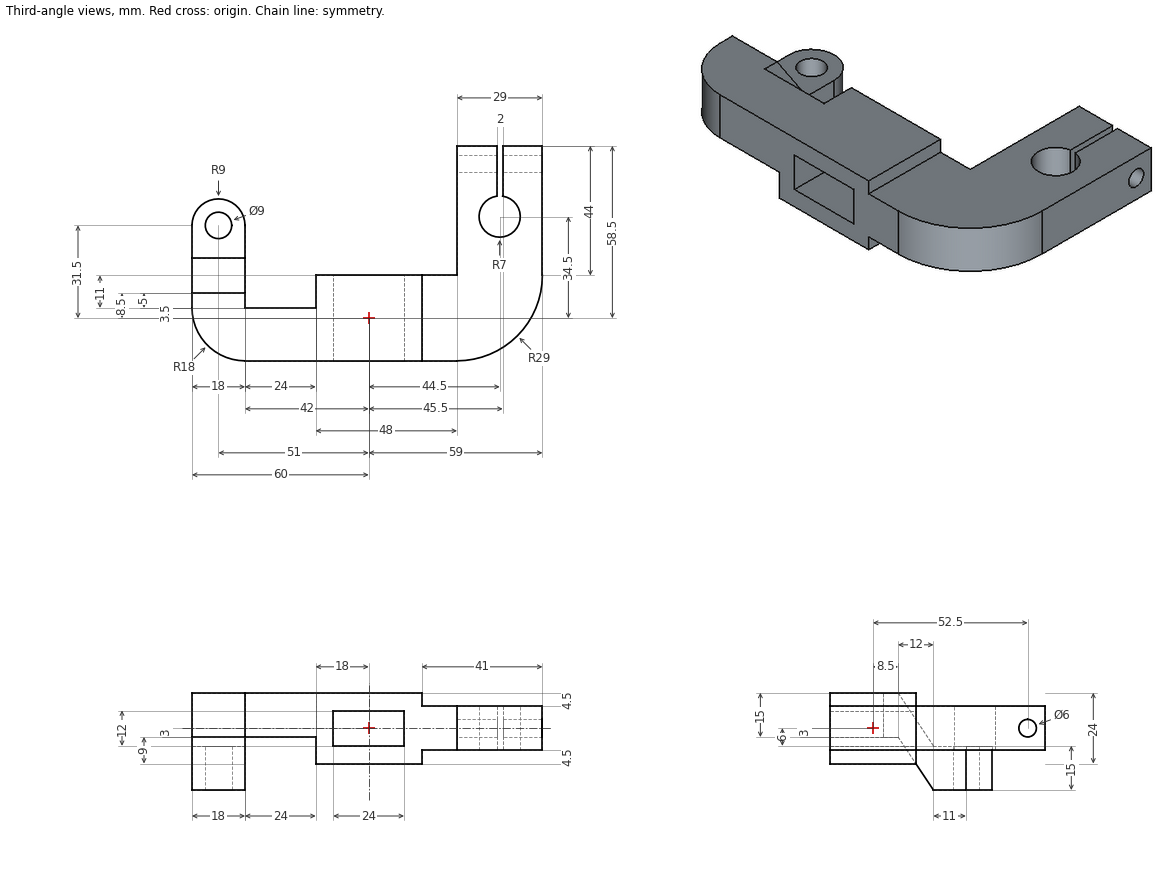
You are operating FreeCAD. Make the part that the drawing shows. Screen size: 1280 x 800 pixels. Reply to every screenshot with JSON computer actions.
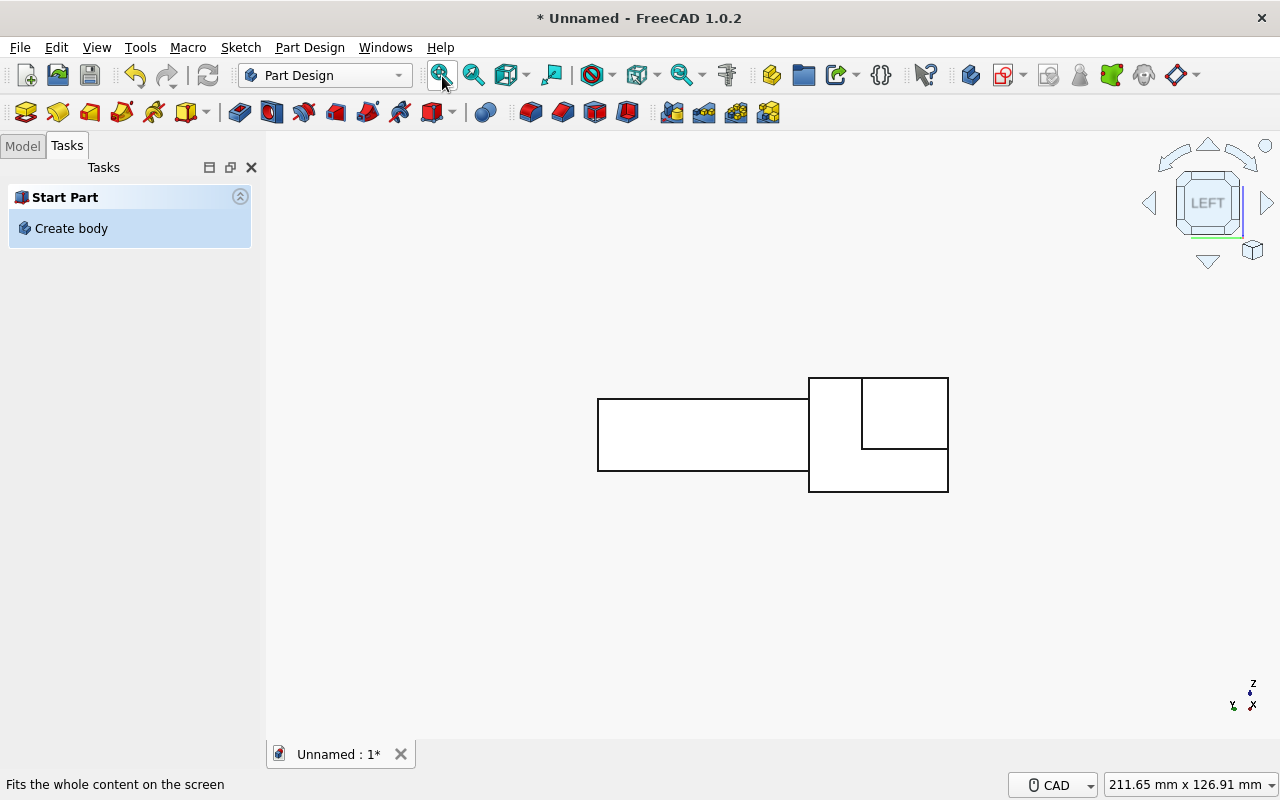
{"action": "left_click", "coordinate": [673, 434]}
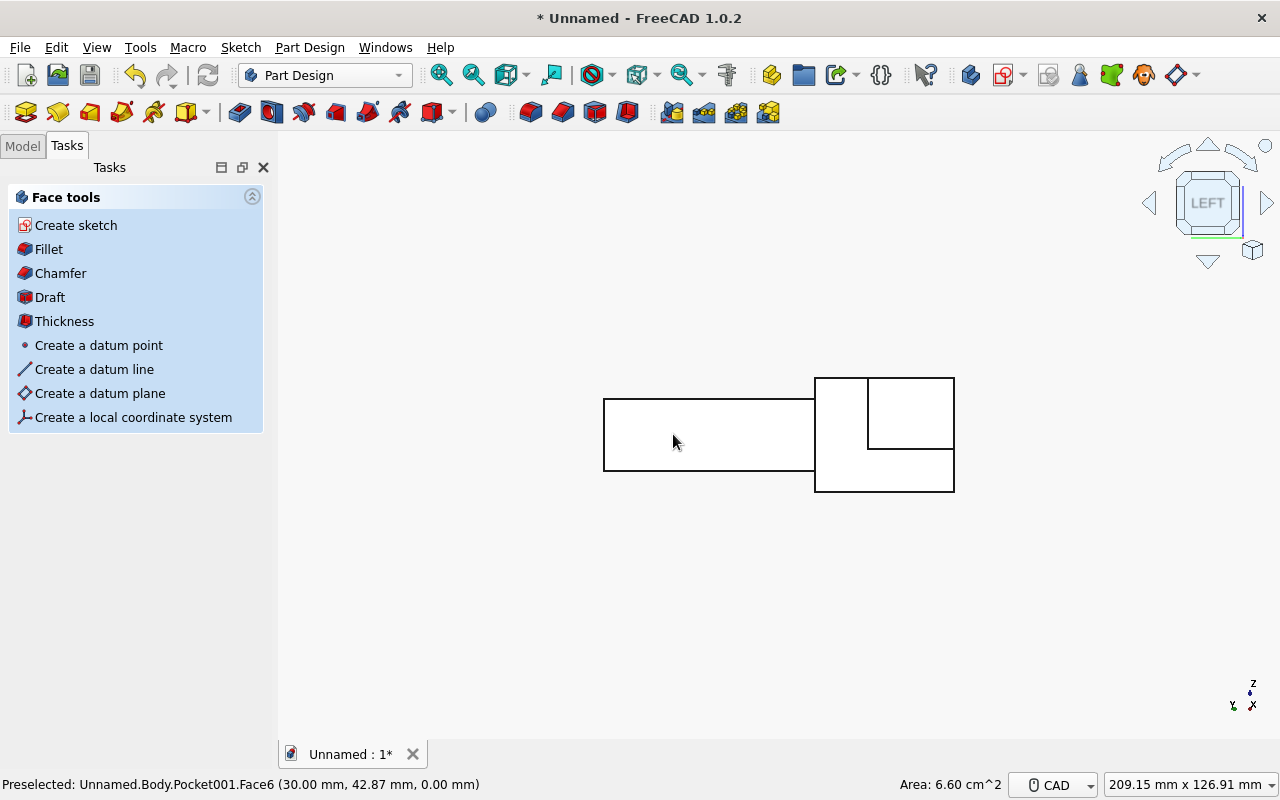
{"action": "left_click", "coordinate": [1004, 76]}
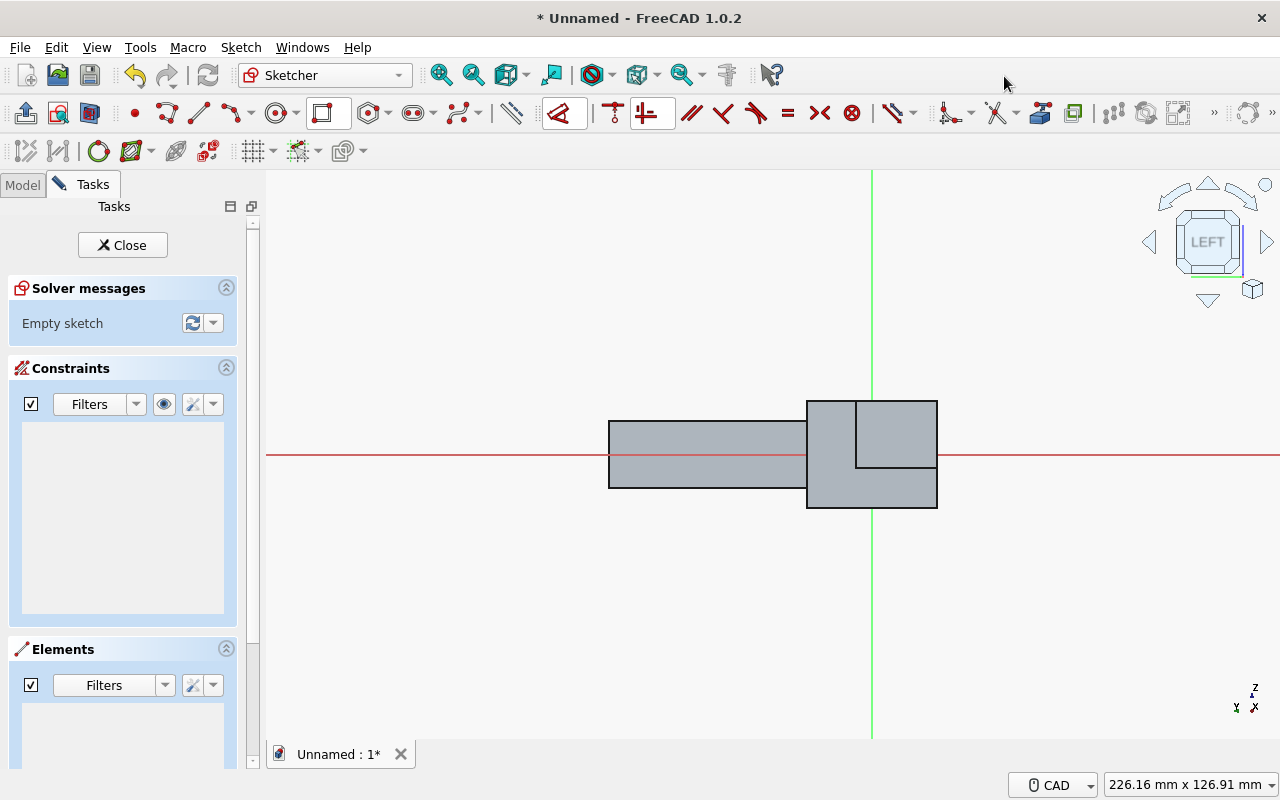
{"action": "scroll", "coordinate": [631, 454], "scroll_direction": "up", "scroll_amount": 13}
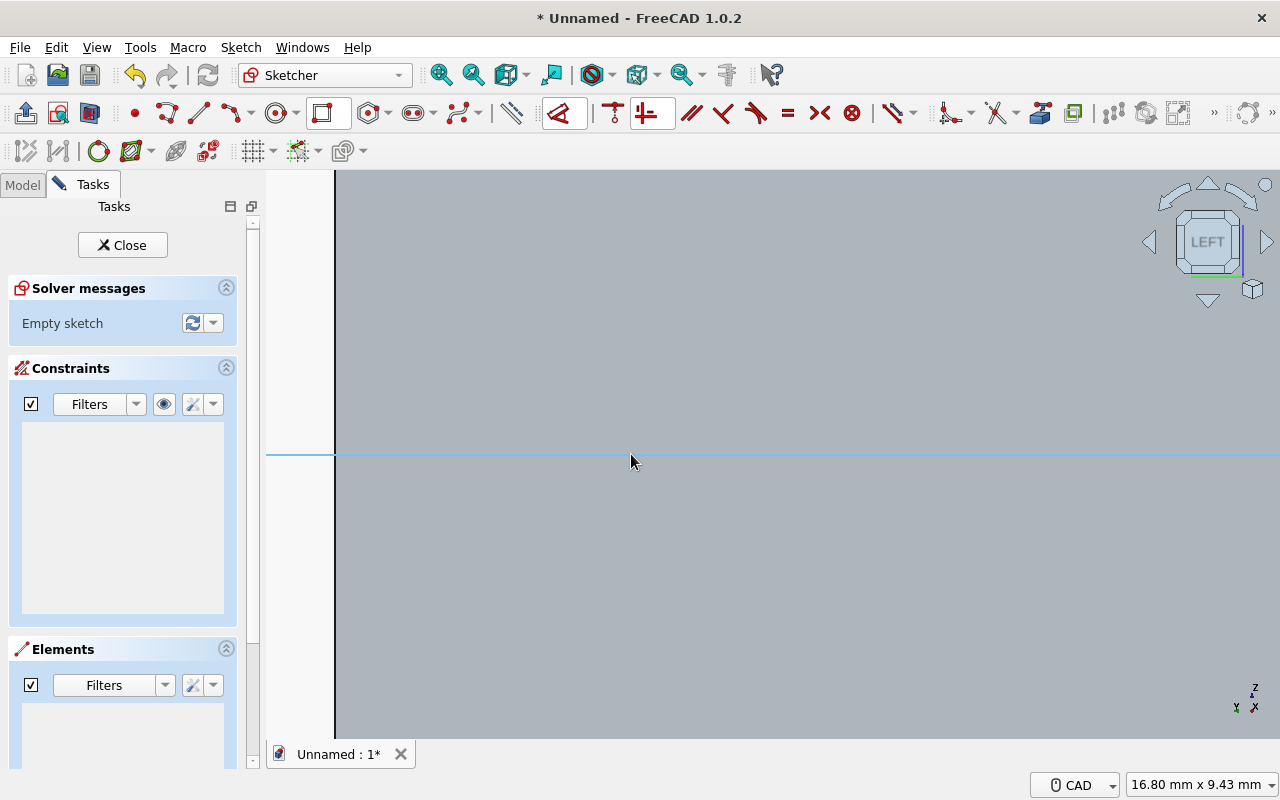
{"action": "left_click", "coordinate": [276, 114]}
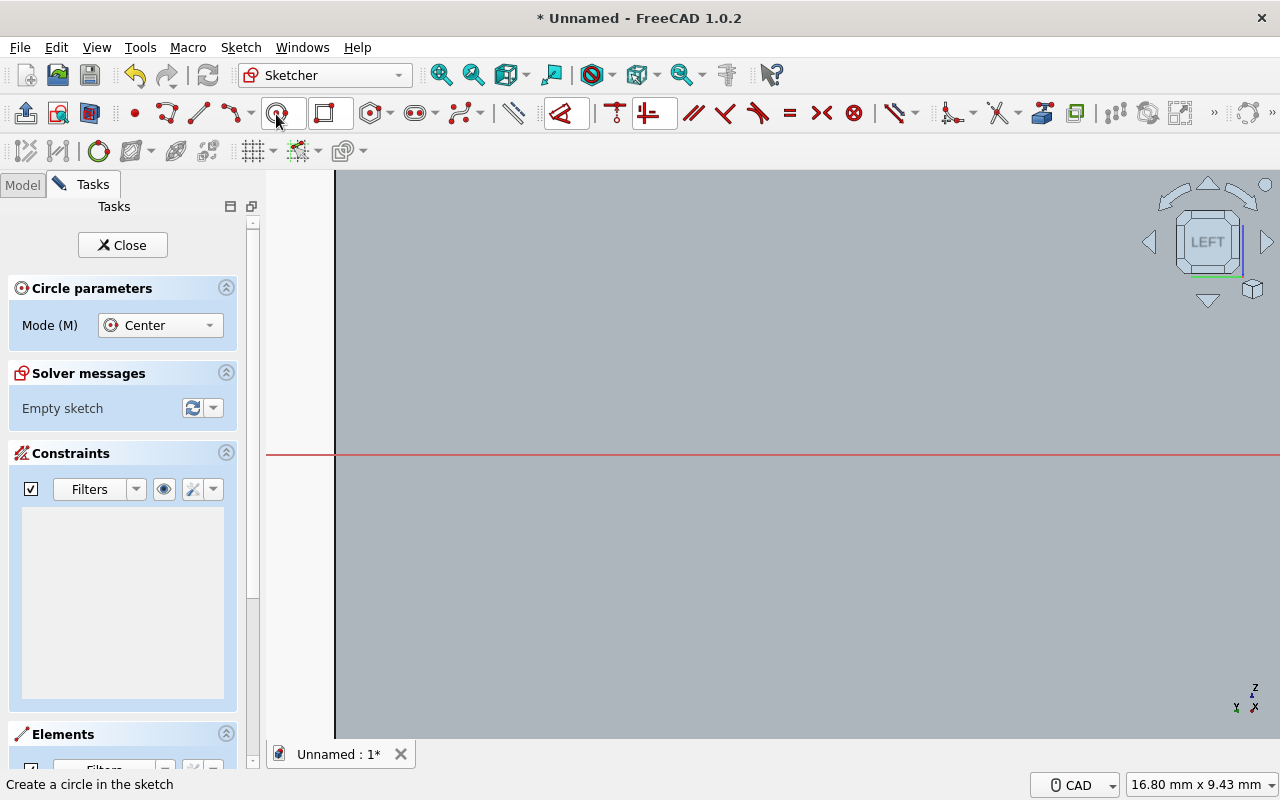
{"action": "left_click", "coordinate": [697, 454]}
{"action": "mouse_move", "coordinate": [825, 326]}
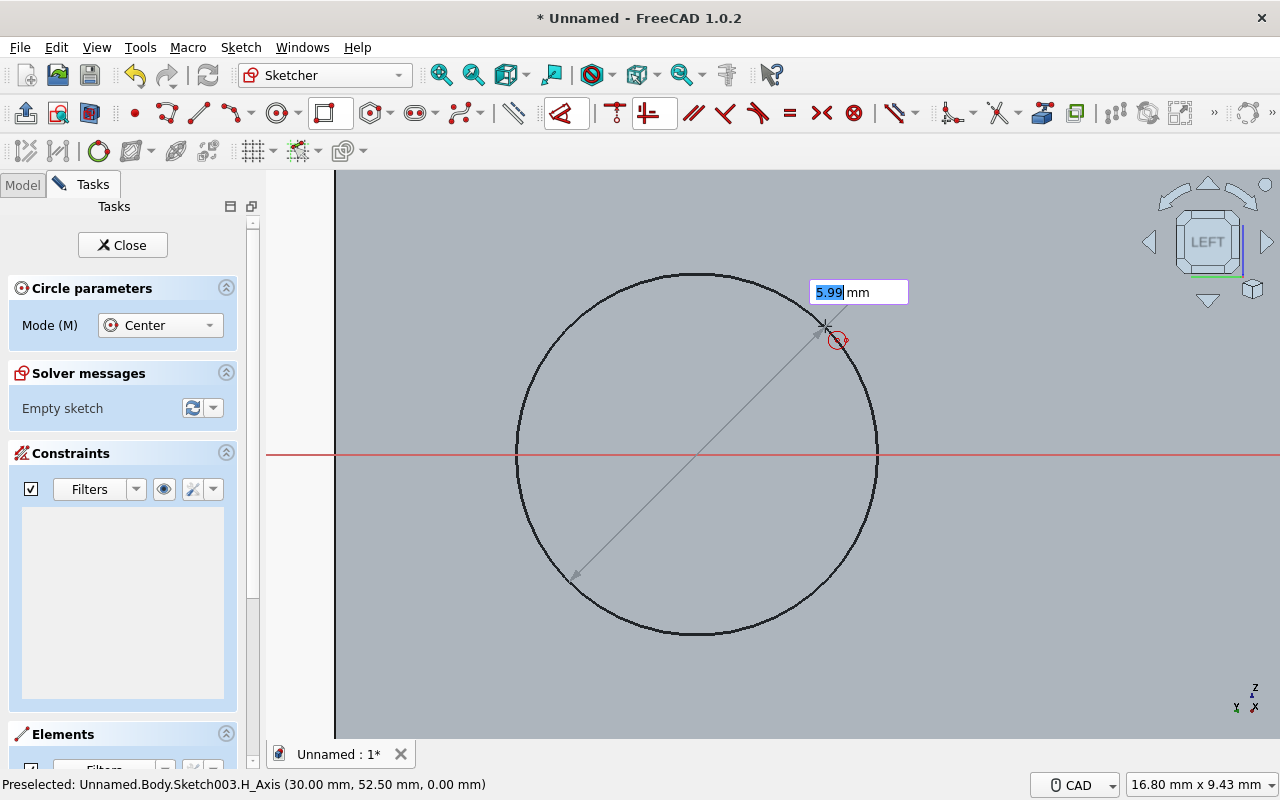
{"action": "type", "text": "6"}
{"action": "key", "text": "Return"}
{"action": "key", "text": "Escape"}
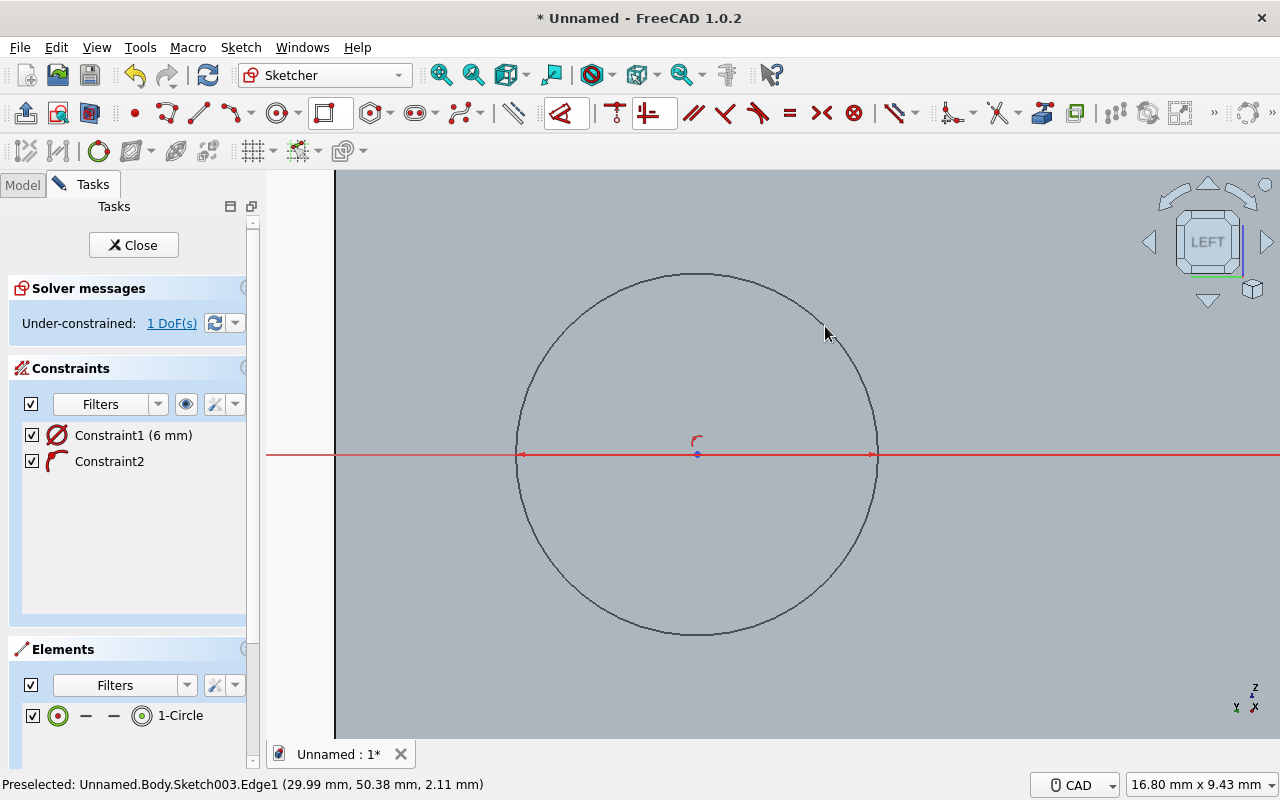
{"action": "left_click", "coordinate": [697, 454]}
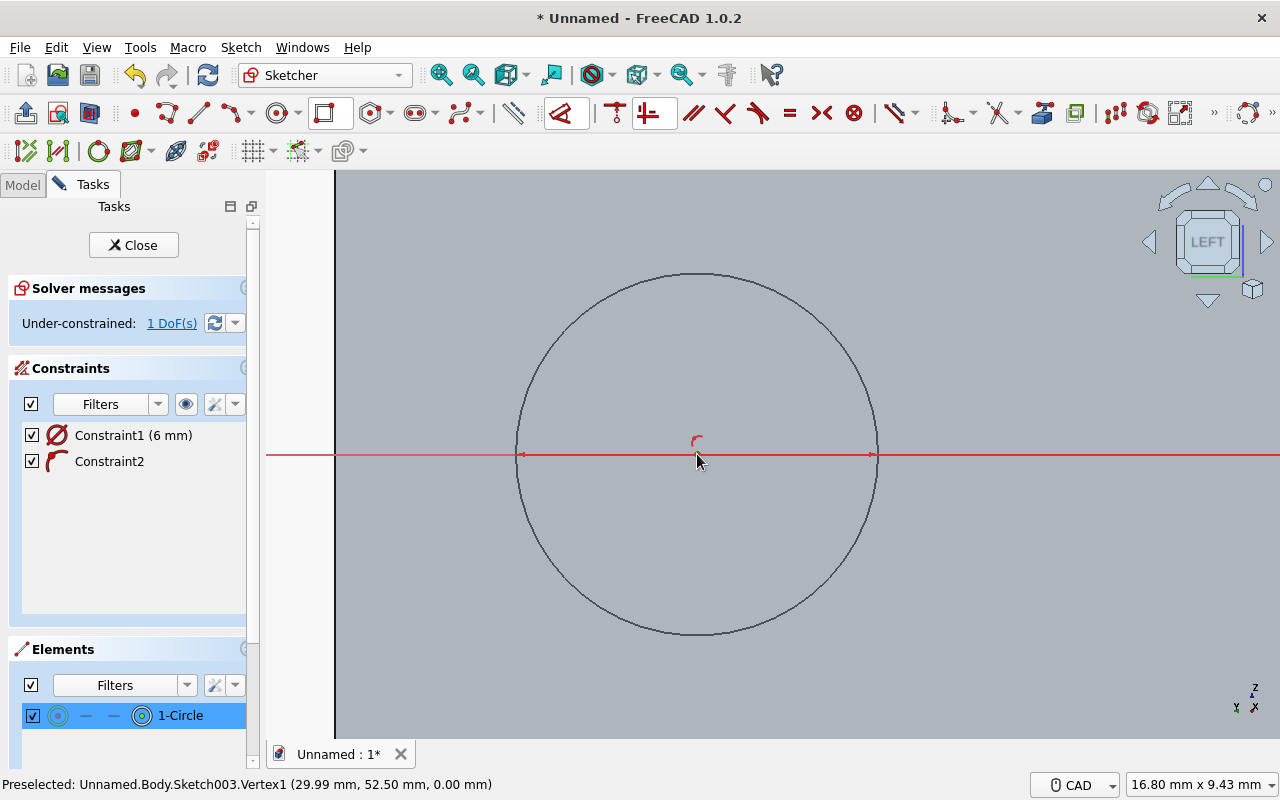
{"action": "key", "text": "l"}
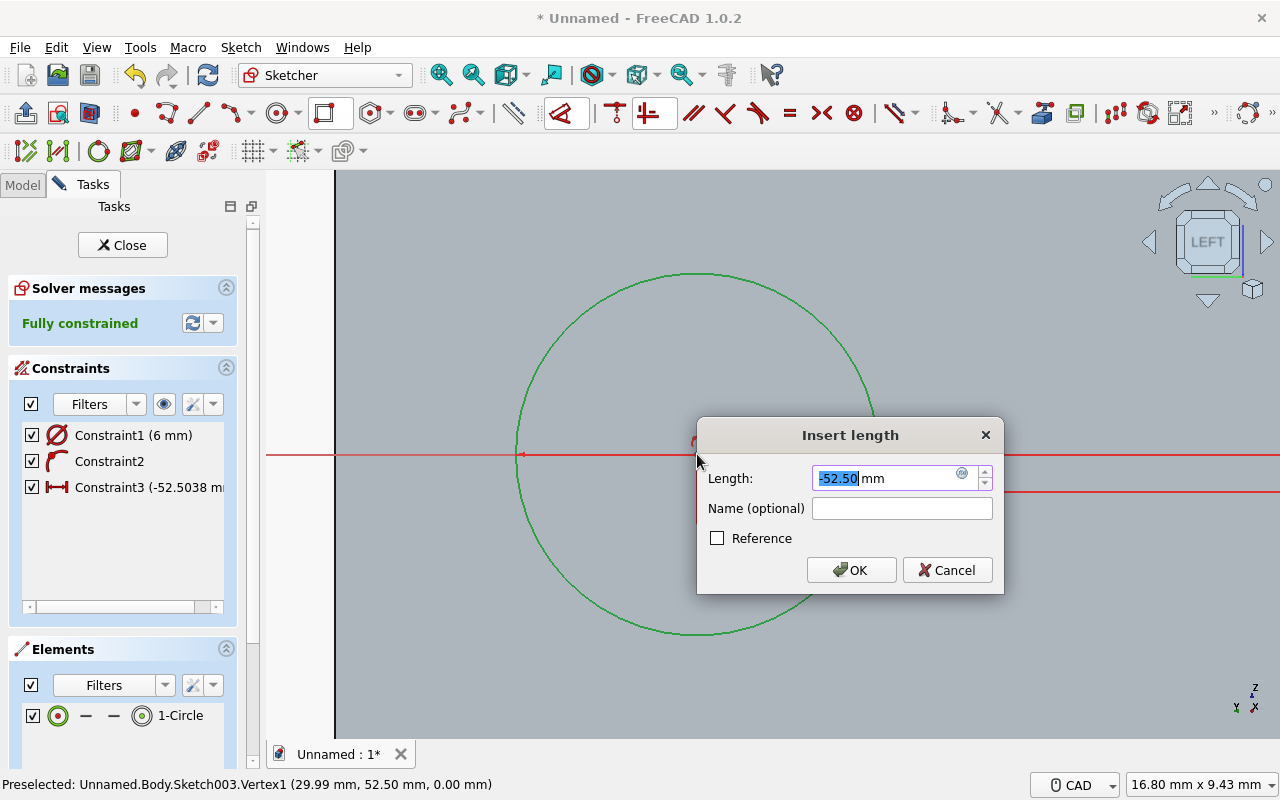
{"action": "type", "text": "-52.5"}
{"action": "key", "text": "Return"}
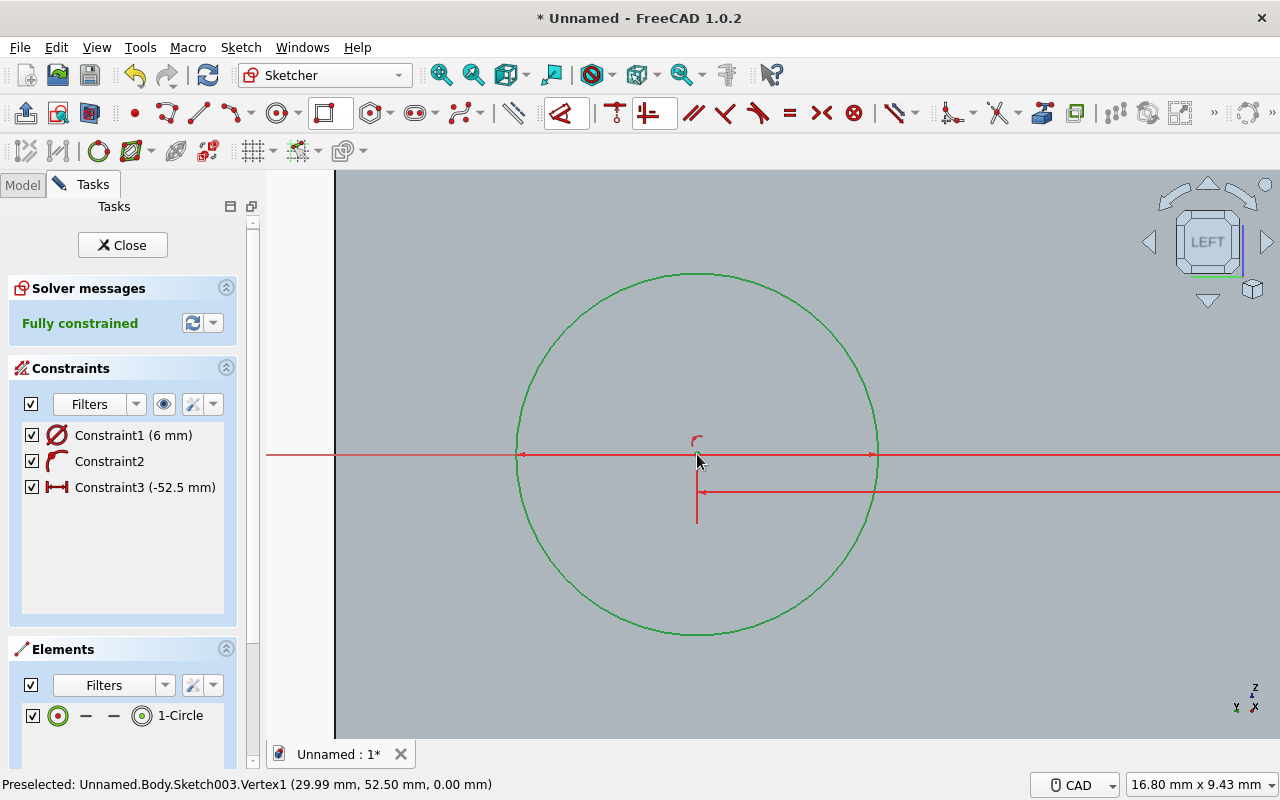
{"action": "left_click", "coordinate": [123, 245]}